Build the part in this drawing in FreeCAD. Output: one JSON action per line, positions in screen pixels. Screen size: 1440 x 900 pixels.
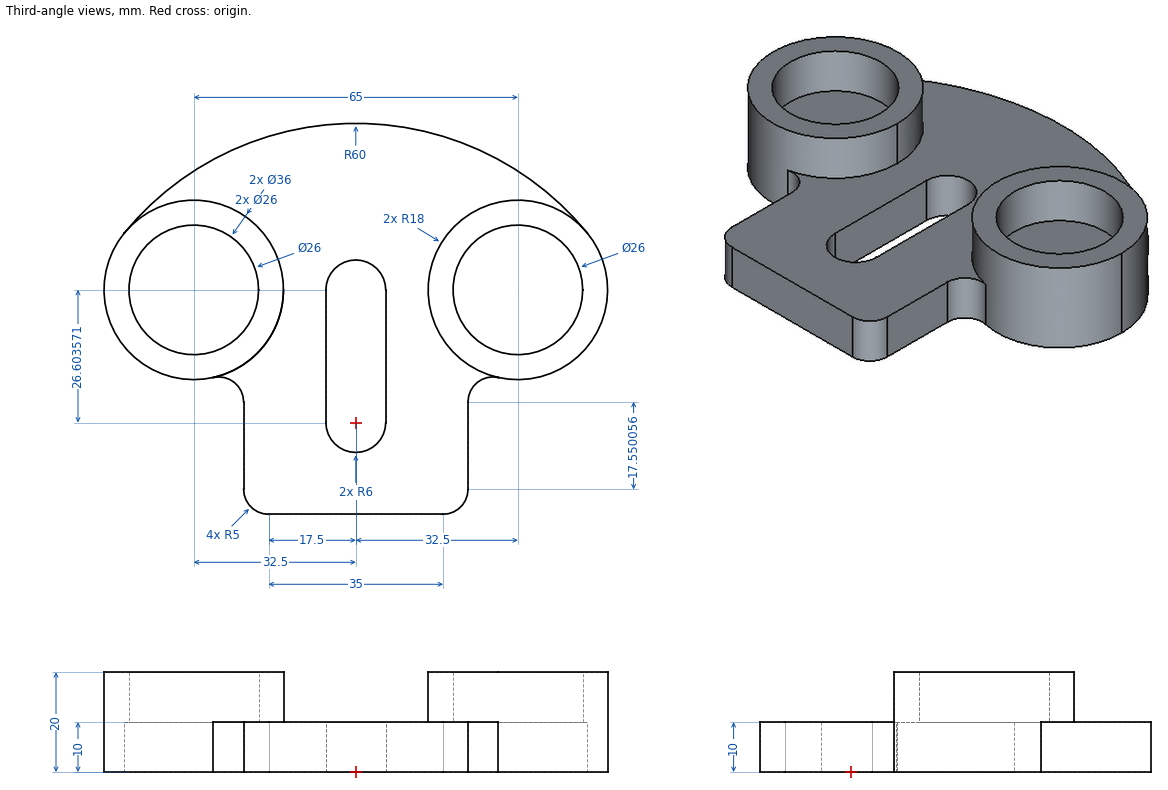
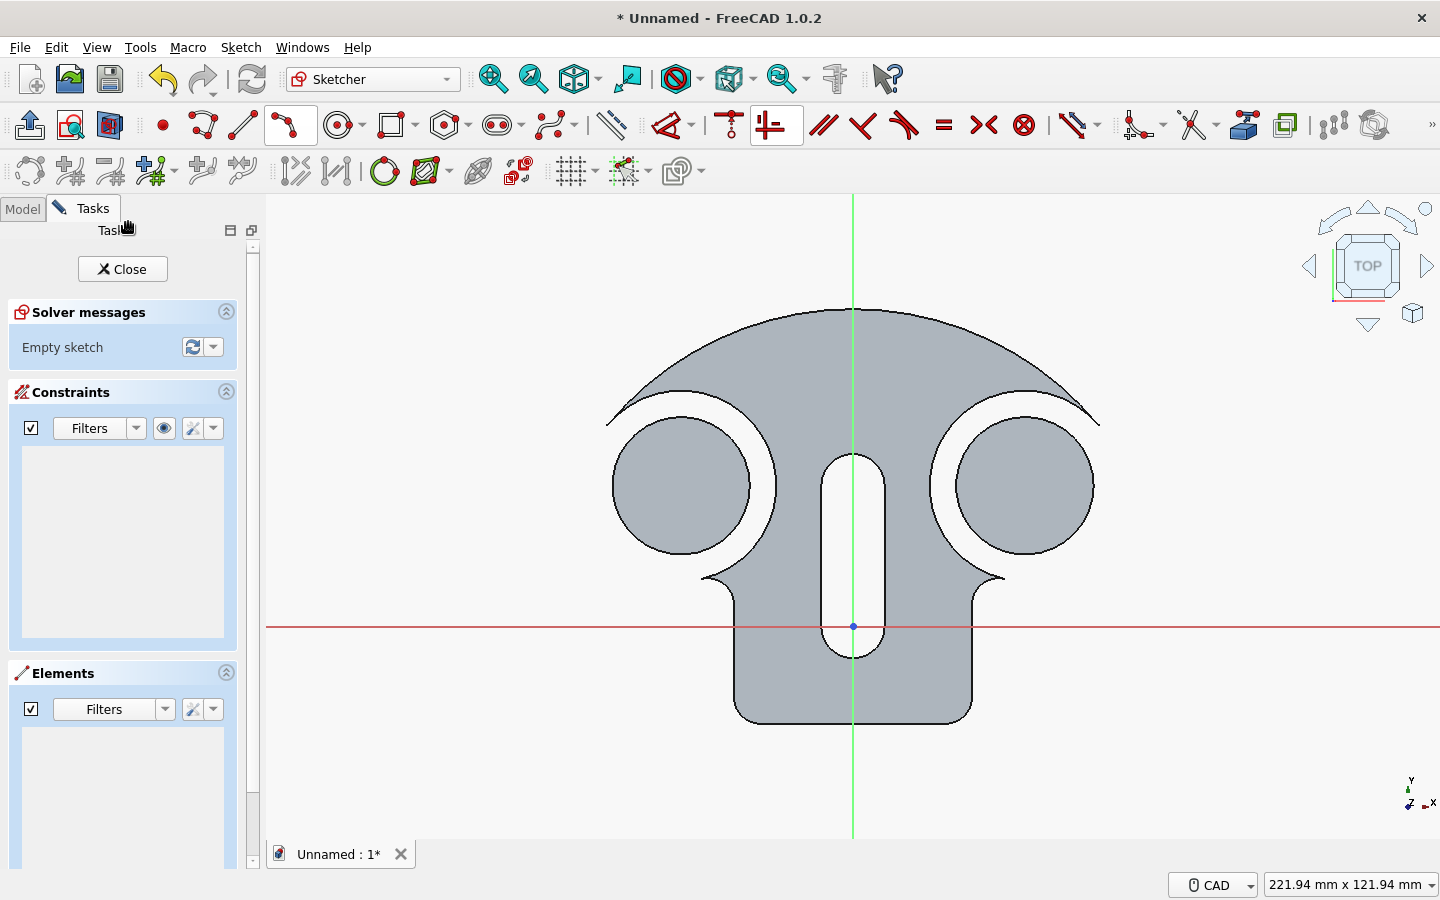
{"action": "key", "text": "g c"}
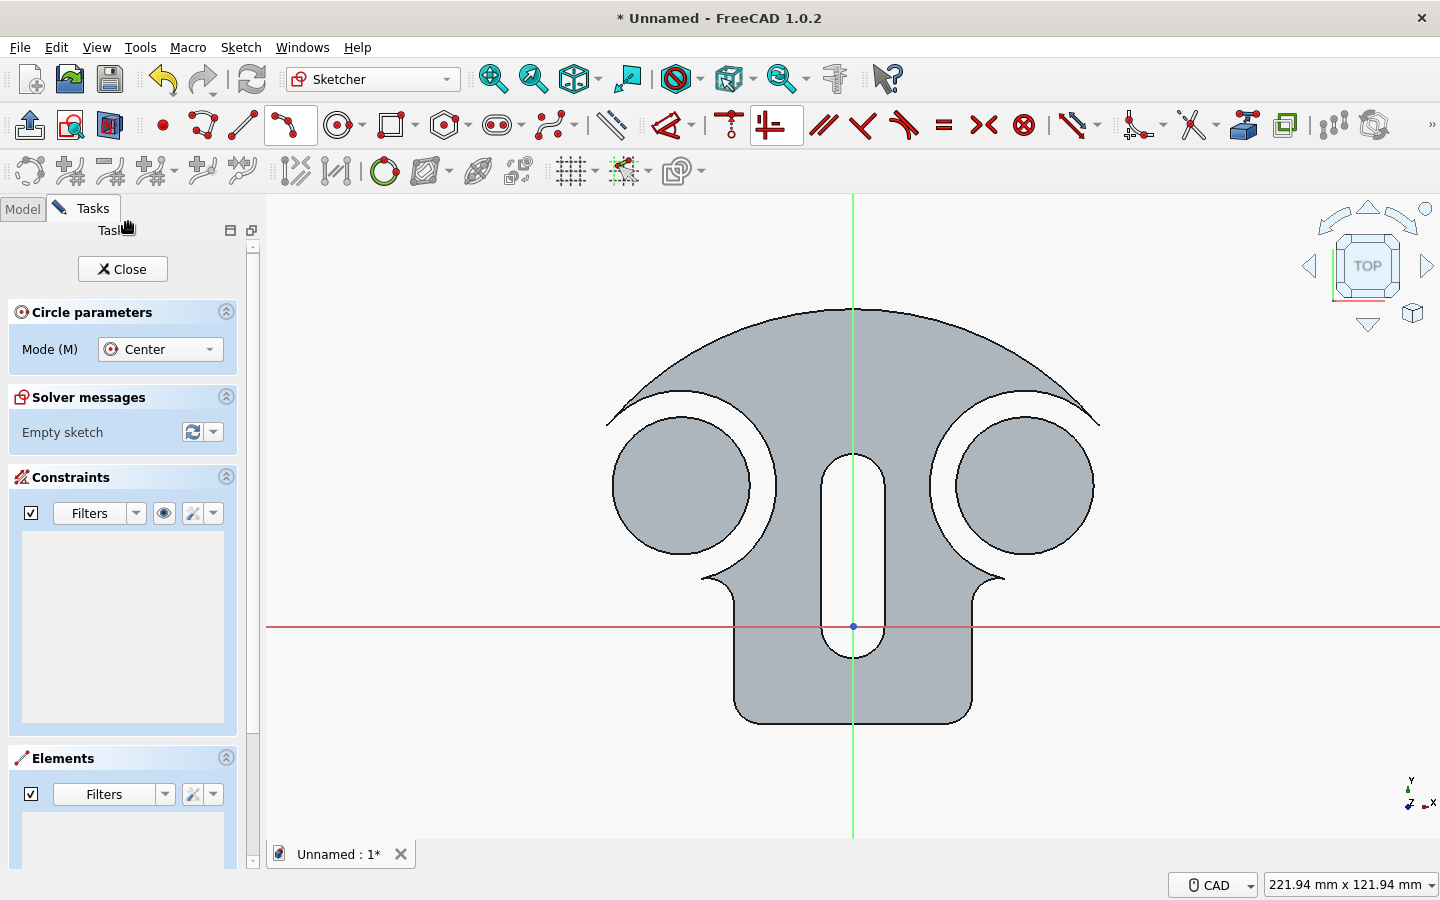
{"action": "left_click", "coordinate": [681, 486]}
{"action": "mouse_move", "coordinate": [748, 418]}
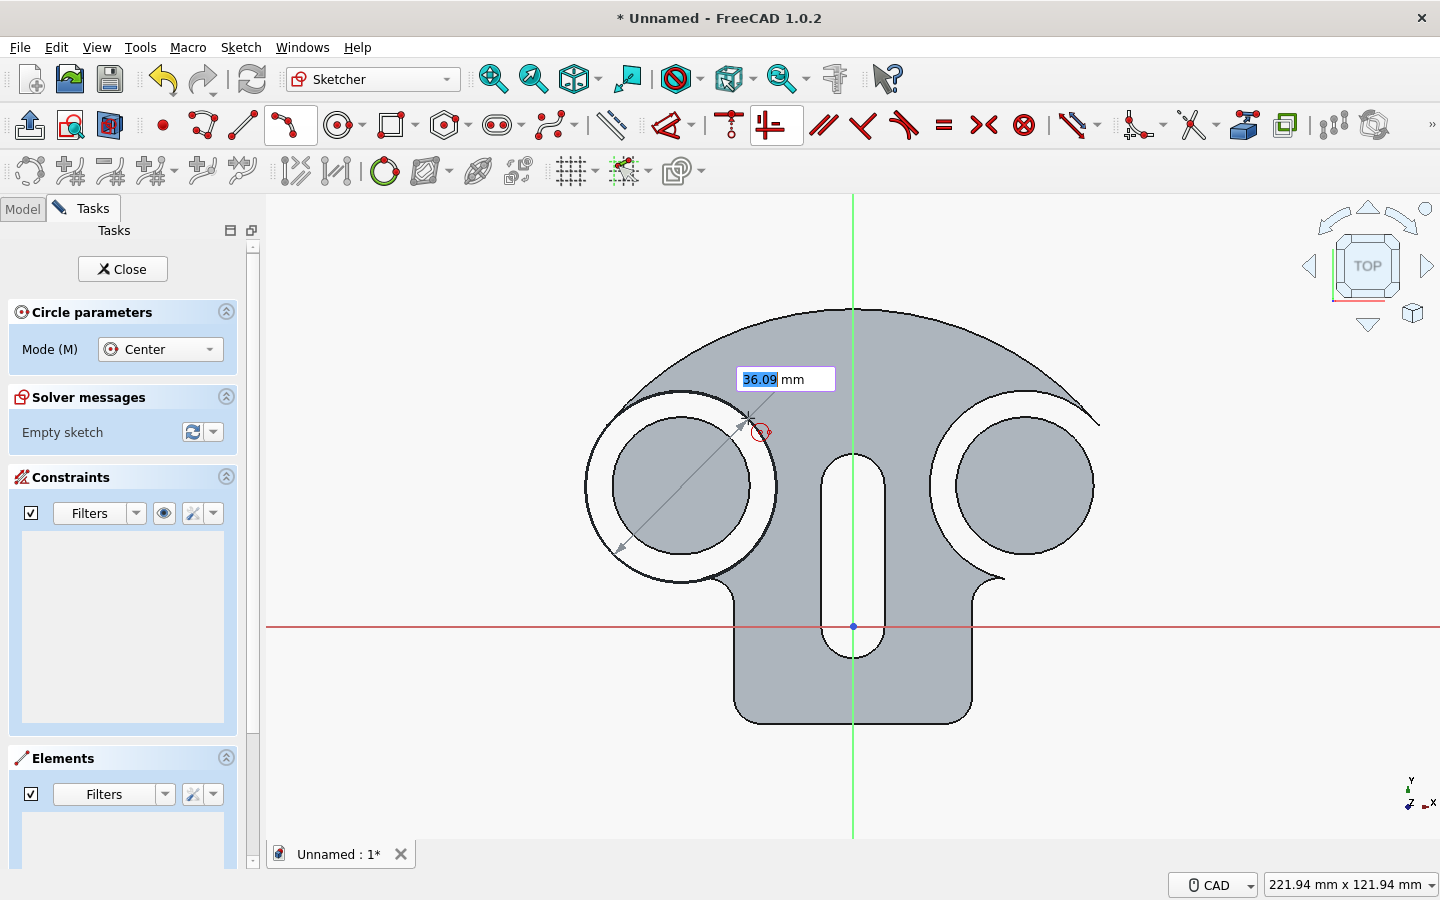
{"action": "type", "text": "36"}
{"action": "key", "text": "Return"}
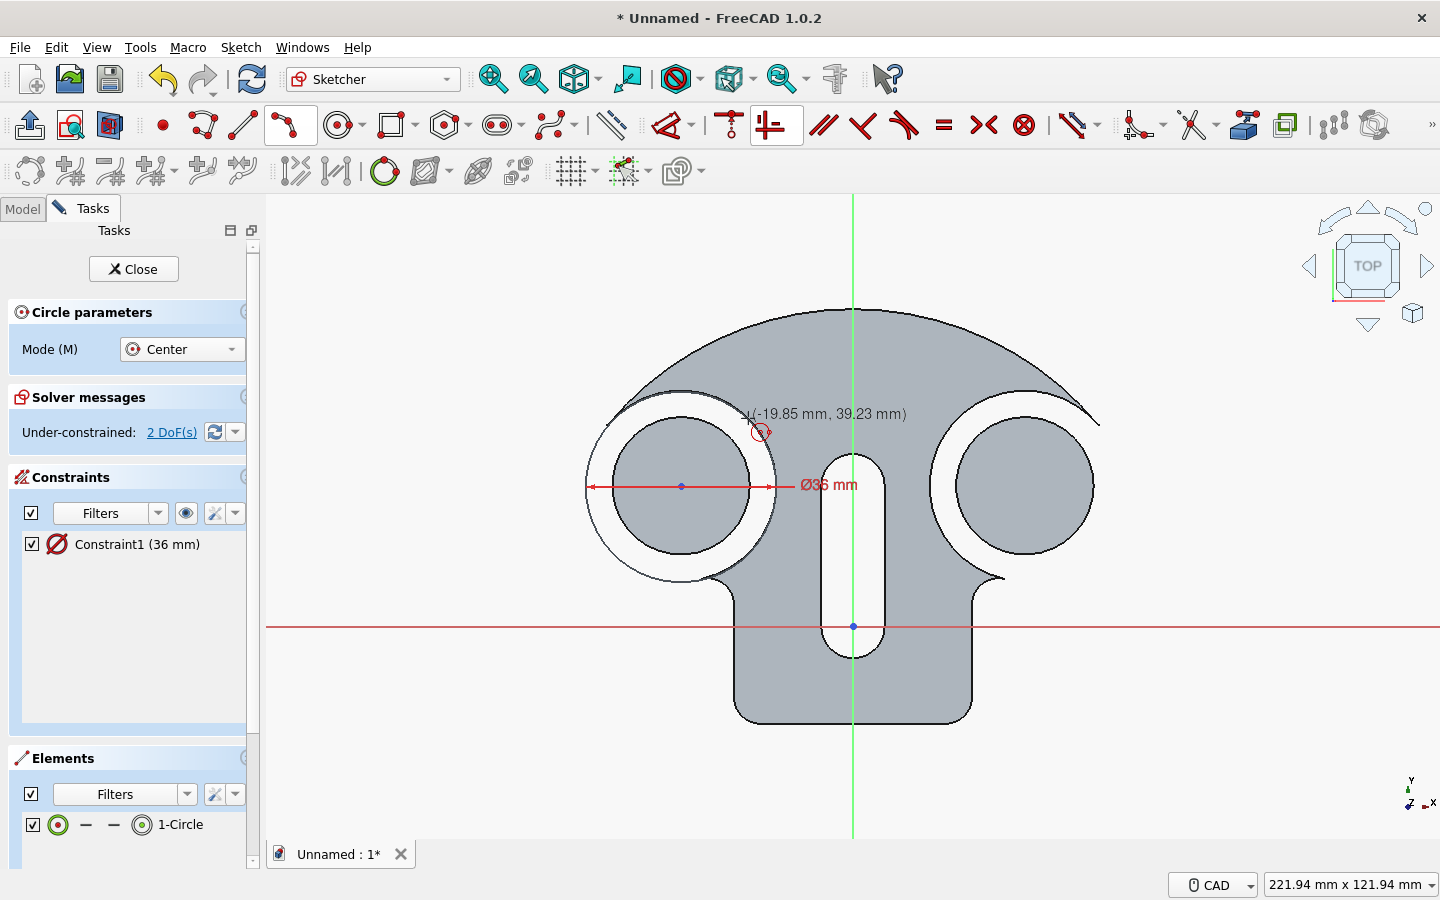
{"action": "left_click", "coordinate": [1025, 486]}
{"action": "mouse_move", "coordinate": [1092, 418]}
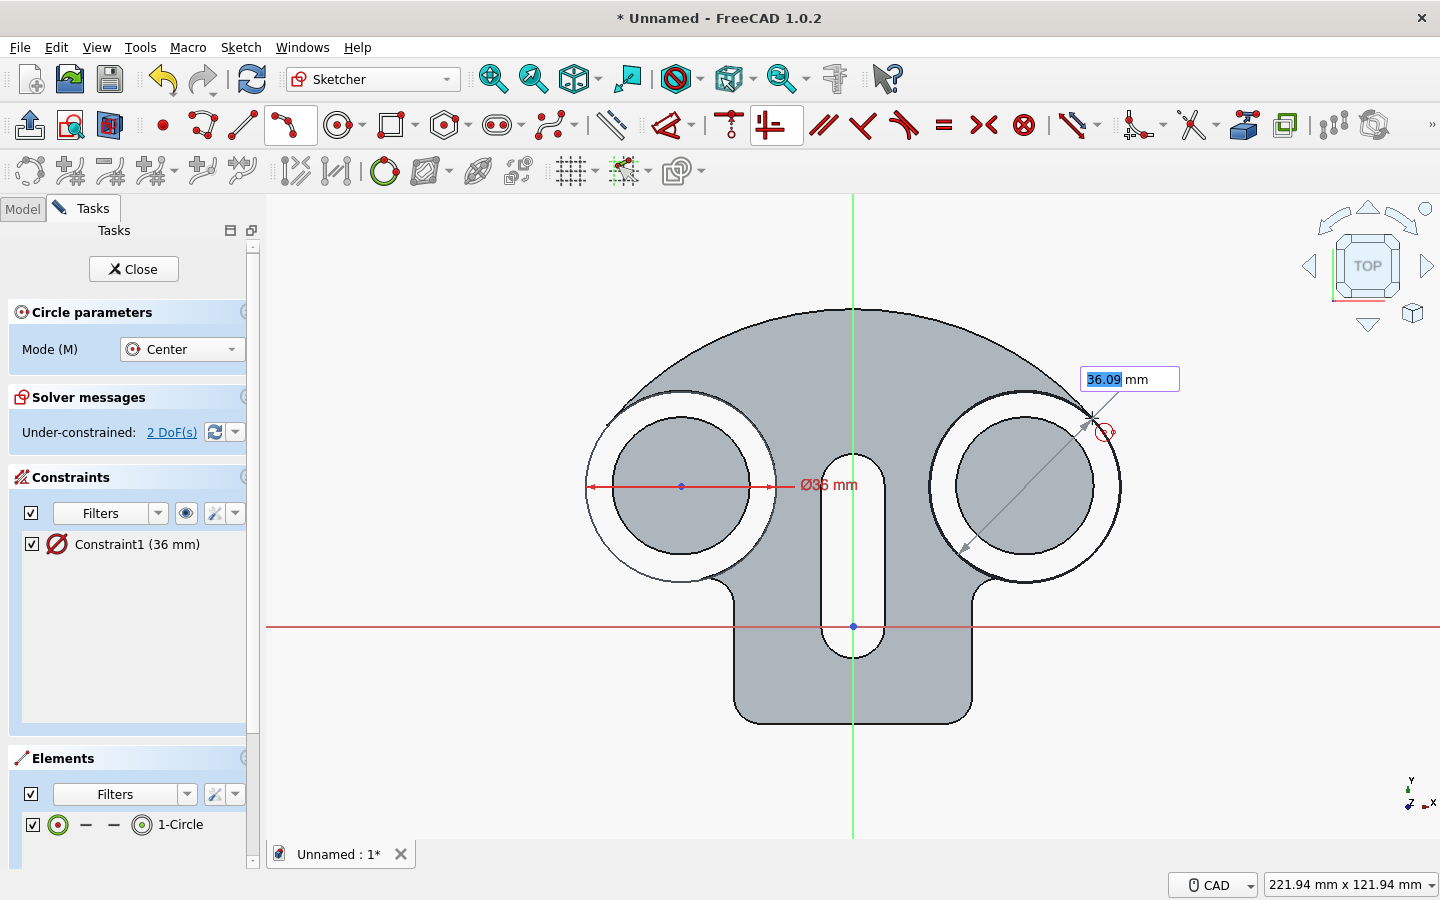
{"action": "type", "text": "36"}
{"action": "key", "text": "Return"}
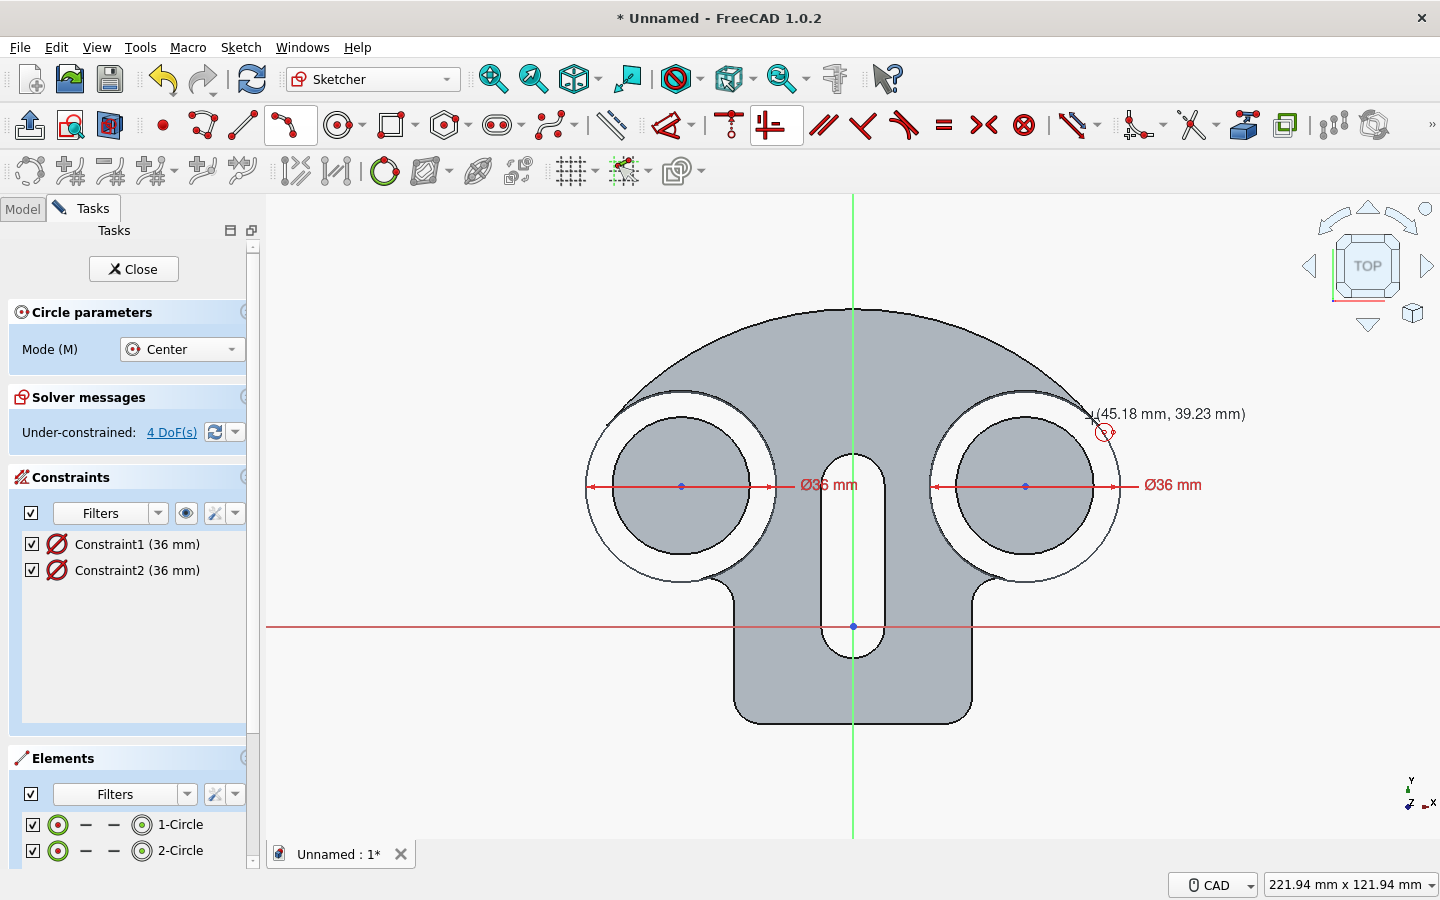
{"action": "left_click", "coordinate": [681, 487]}
{"action": "mouse_move", "coordinate": [730, 437]}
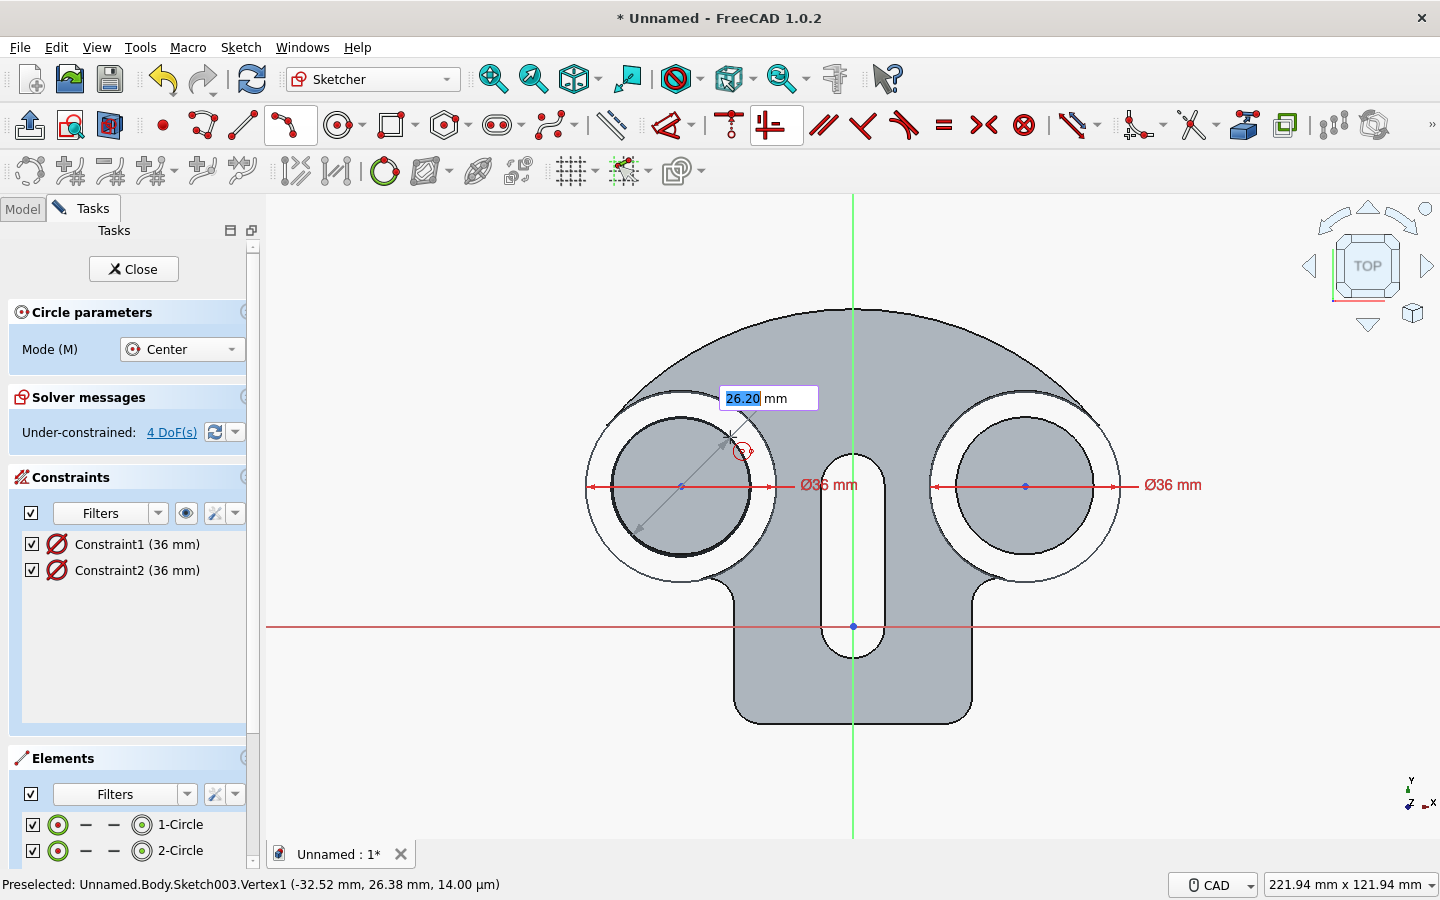
{"action": "type", "text": "26"}
{"action": "key", "text": "Return"}